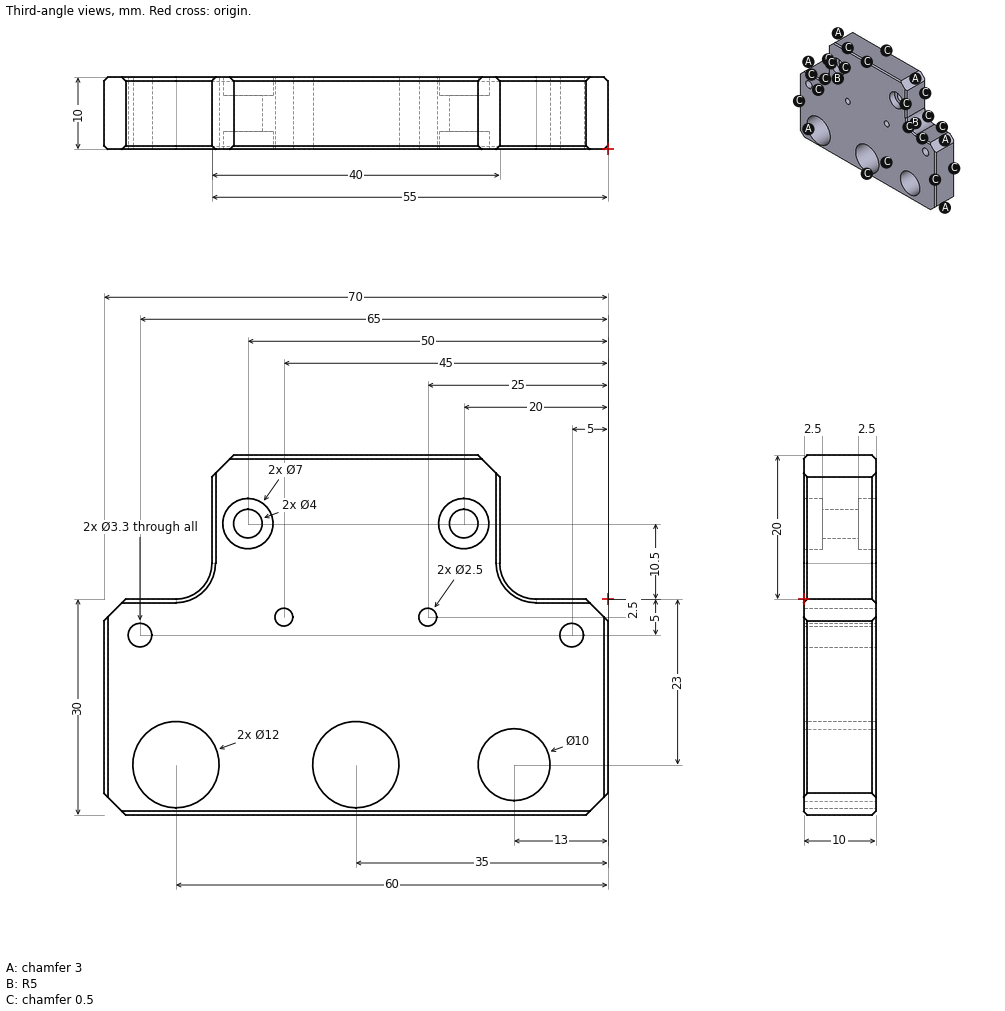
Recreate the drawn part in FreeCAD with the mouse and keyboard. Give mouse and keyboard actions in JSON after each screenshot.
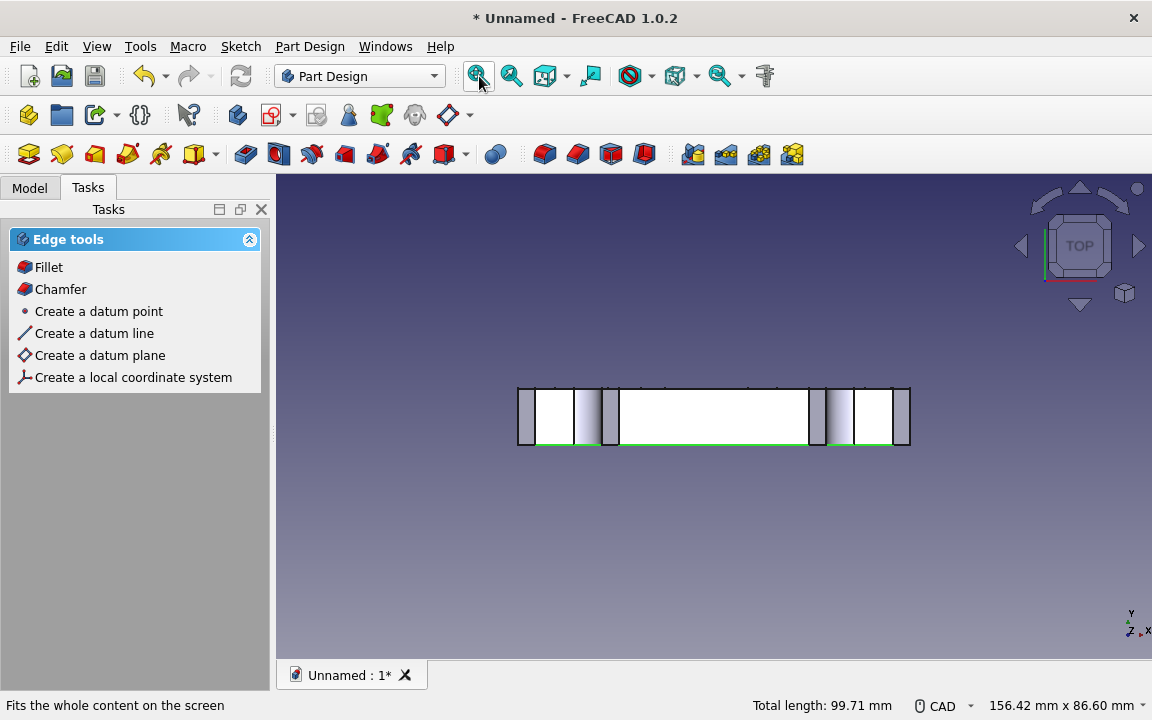
{"action": "left_click", "coordinate": [874, 387], "text": "ctrl"}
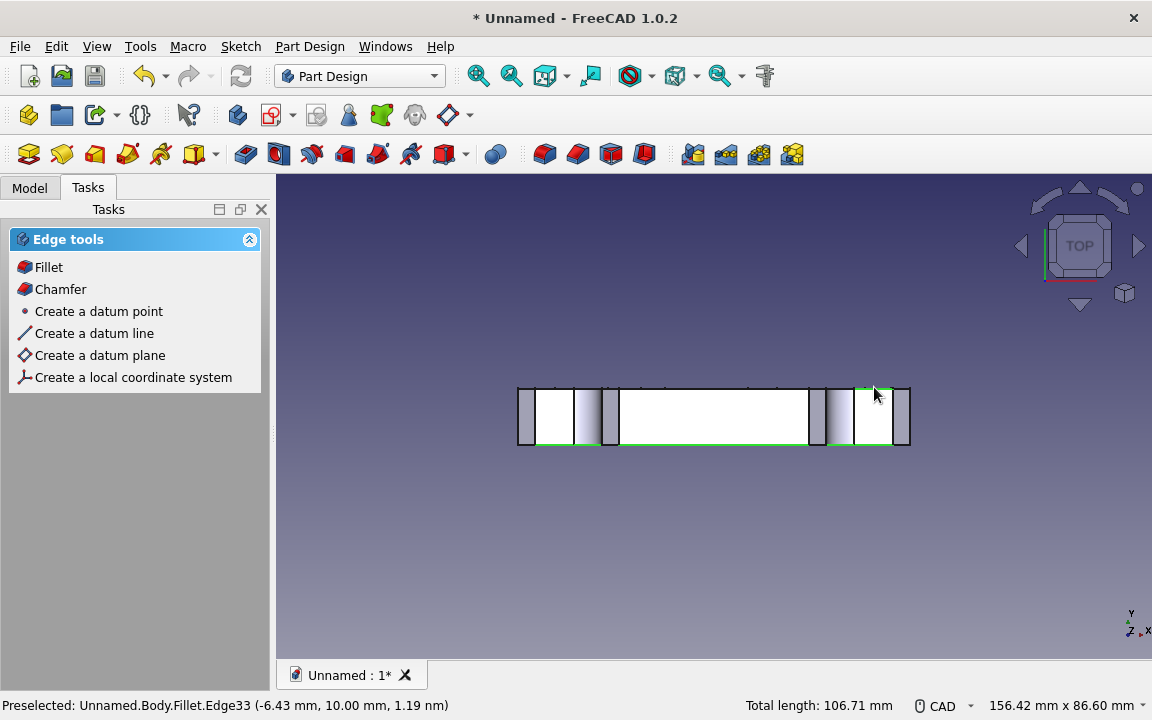
{"action": "left_click", "coordinate": [834, 387], "text": "ctrl"}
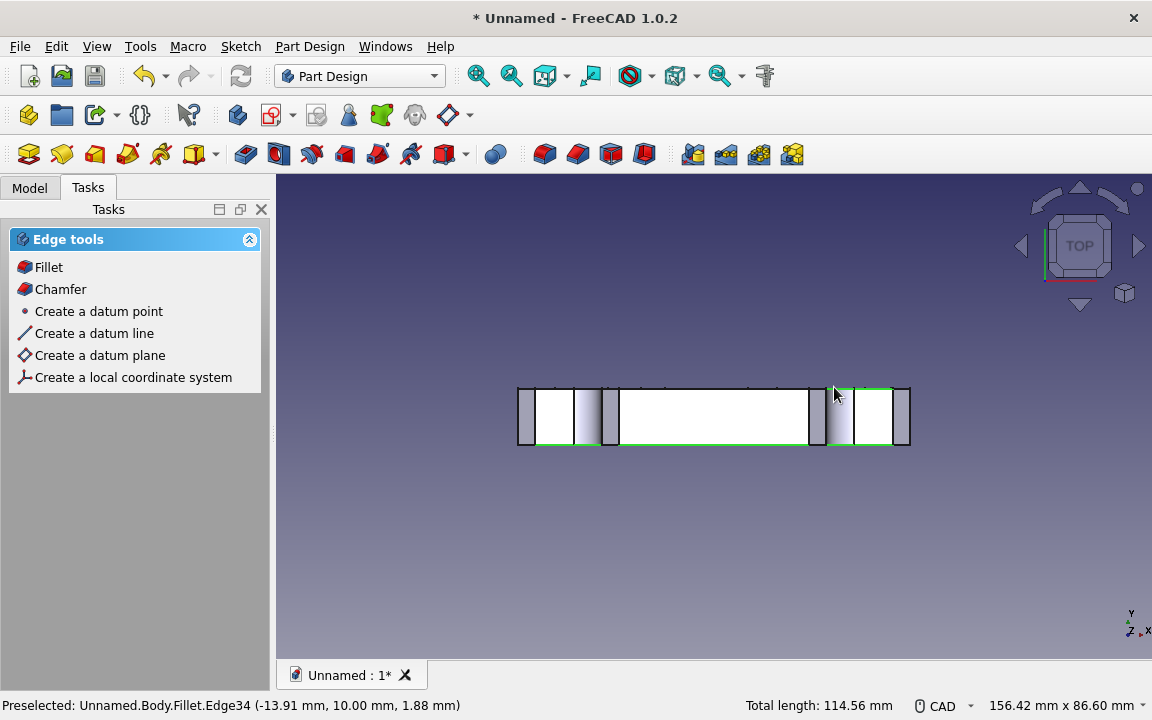
{"action": "left_click", "coordinate": [594, 387], "text": "ctrl"}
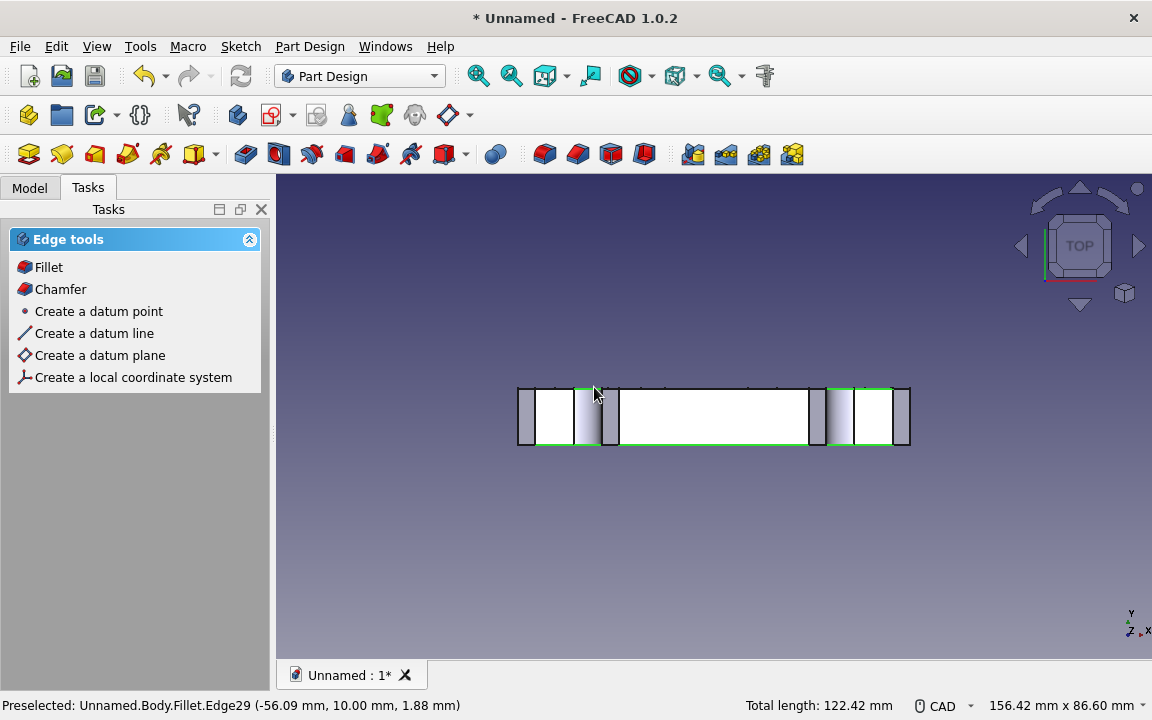
{"action": "left_click", "coordinate": [554, 387], "text": "ctrl"}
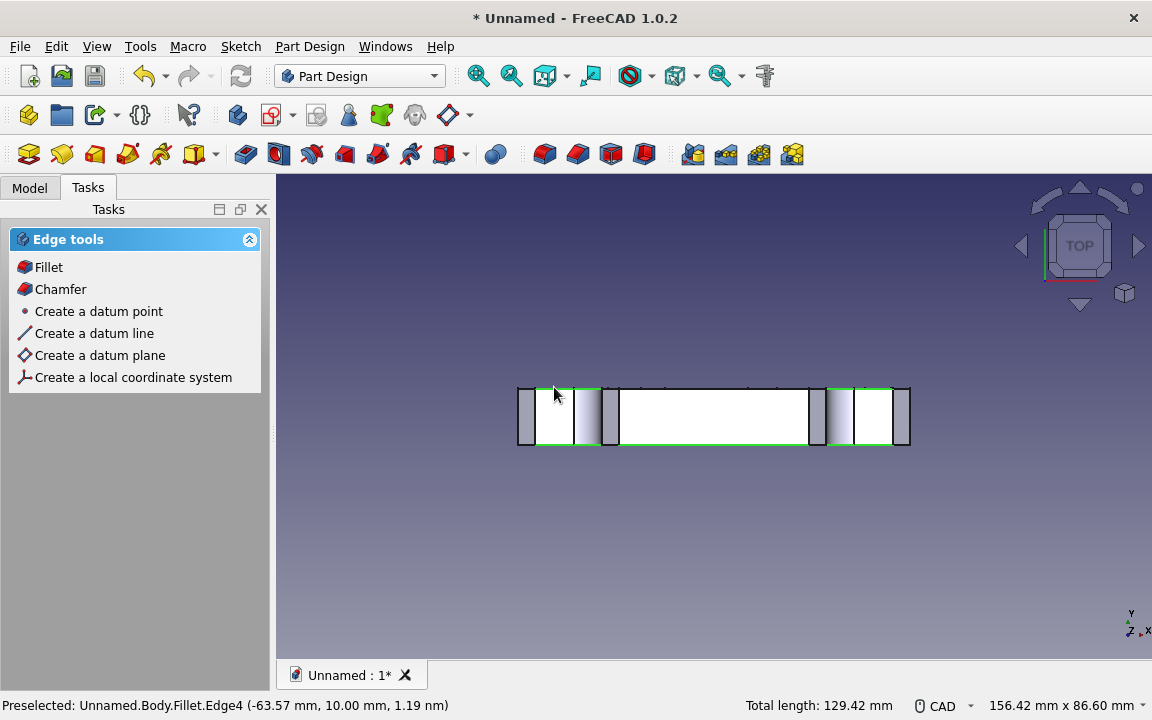
{"action": "left_click", "coordinate": [714, 387], "text": "ctrl"}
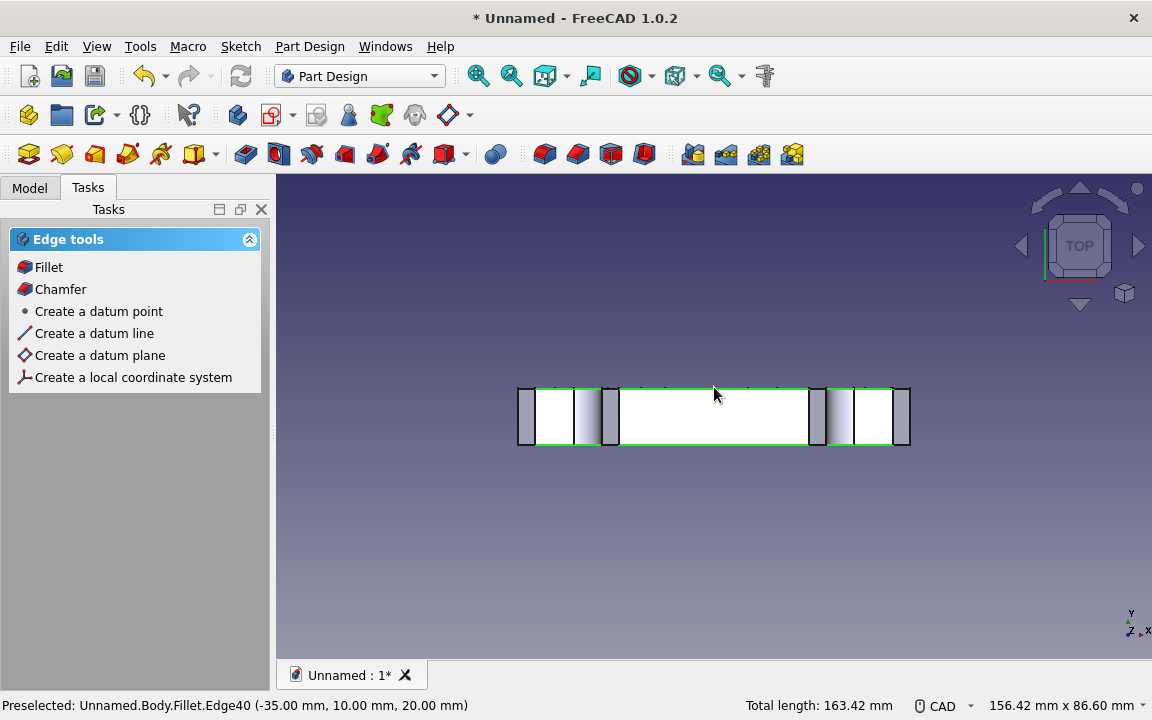
{"action": "key", "text": "0"}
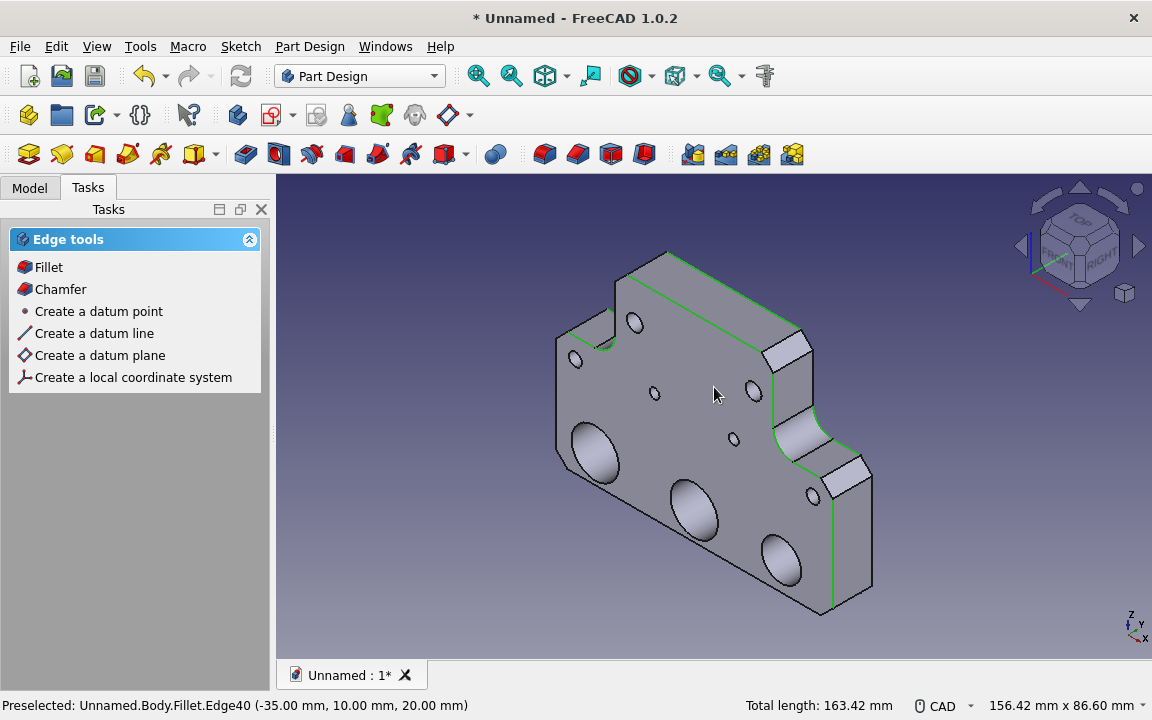
{"action": "key", "text": "1"}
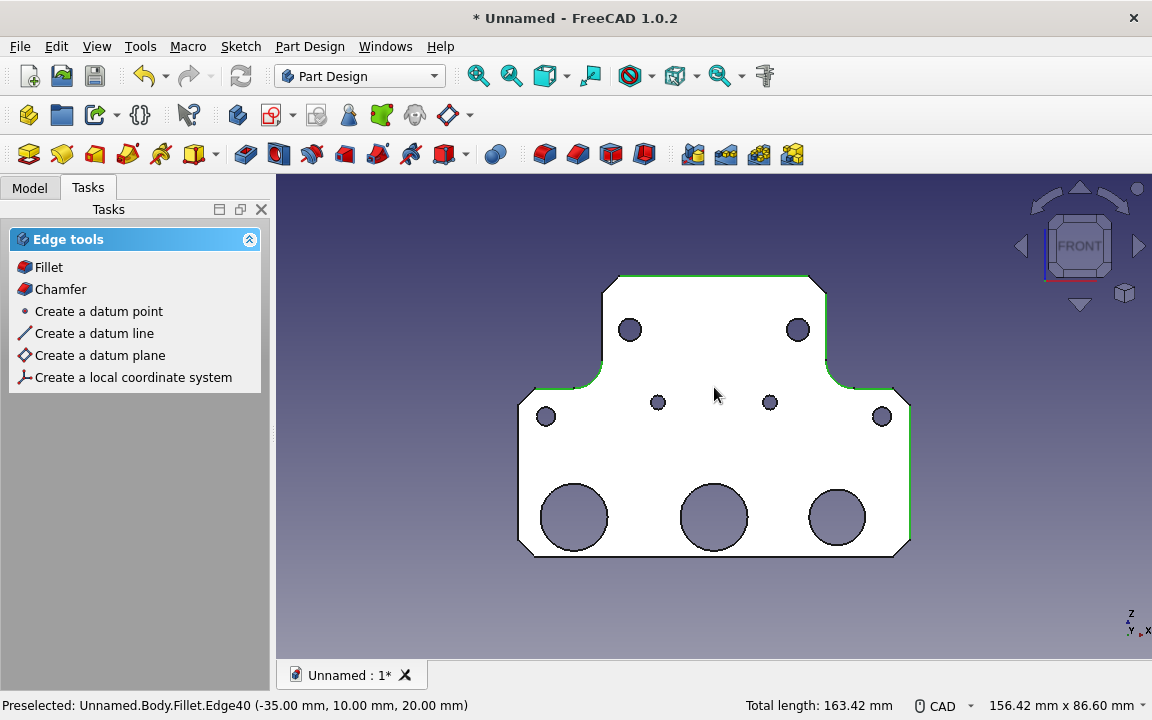
{"action": "left_click", "coordinate": [518, 485], "text": "ctrl"}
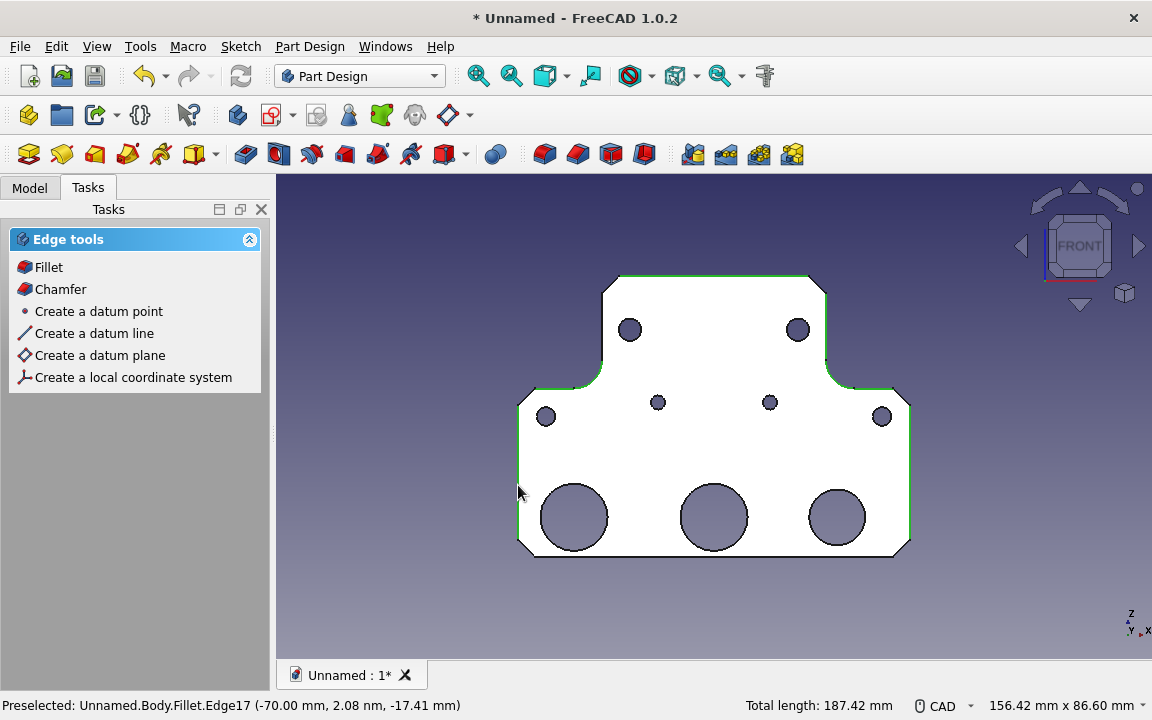
{"action": "key", "text": "3"}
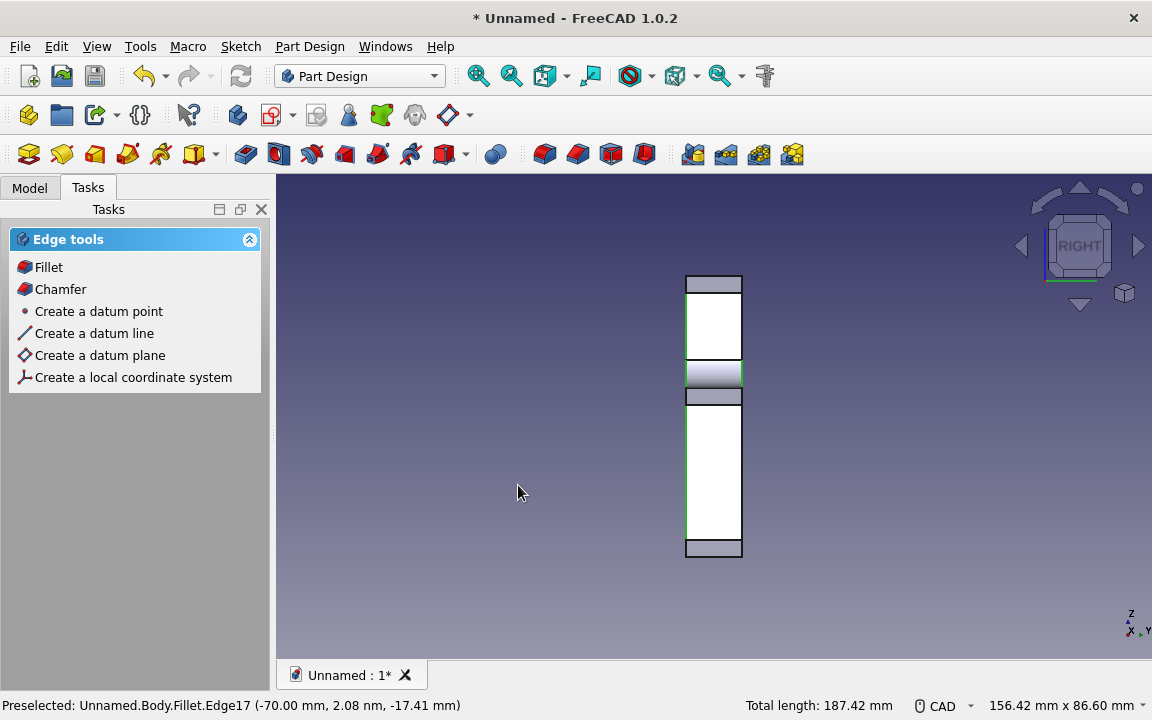
{"action": "left_click", "coordinate": [742, 458], "text": "ctrl"}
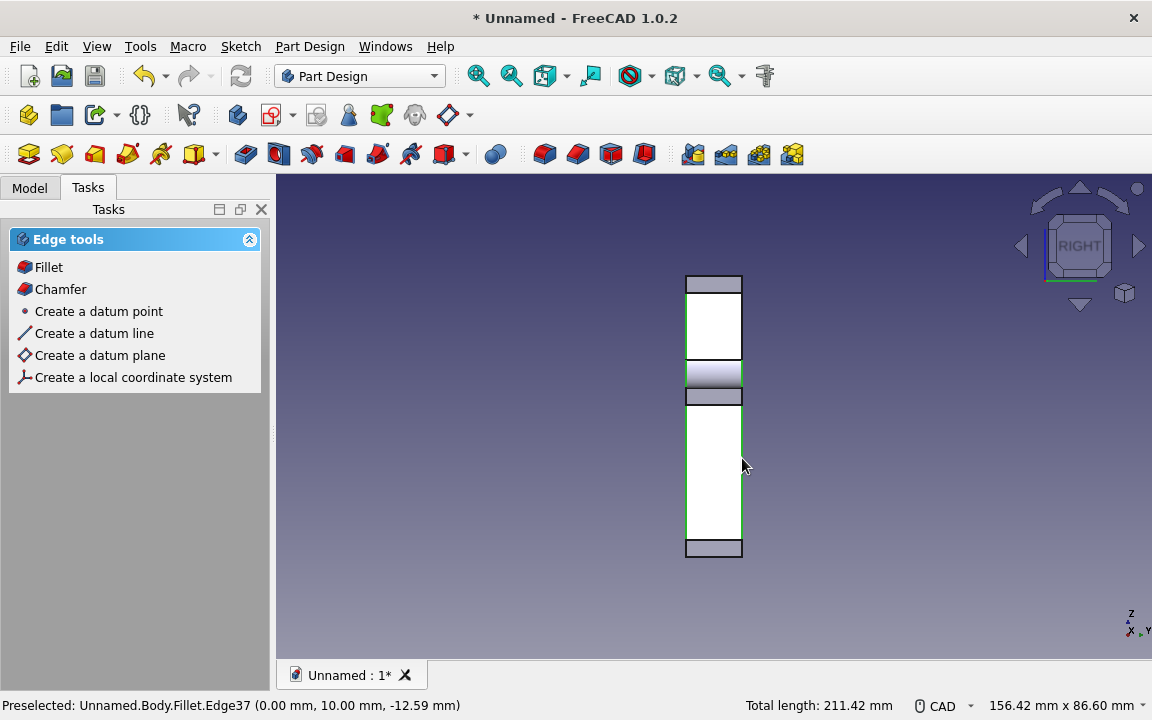
{"action": "left_click", "coordinate": [742, 326], "text": "ctrl"}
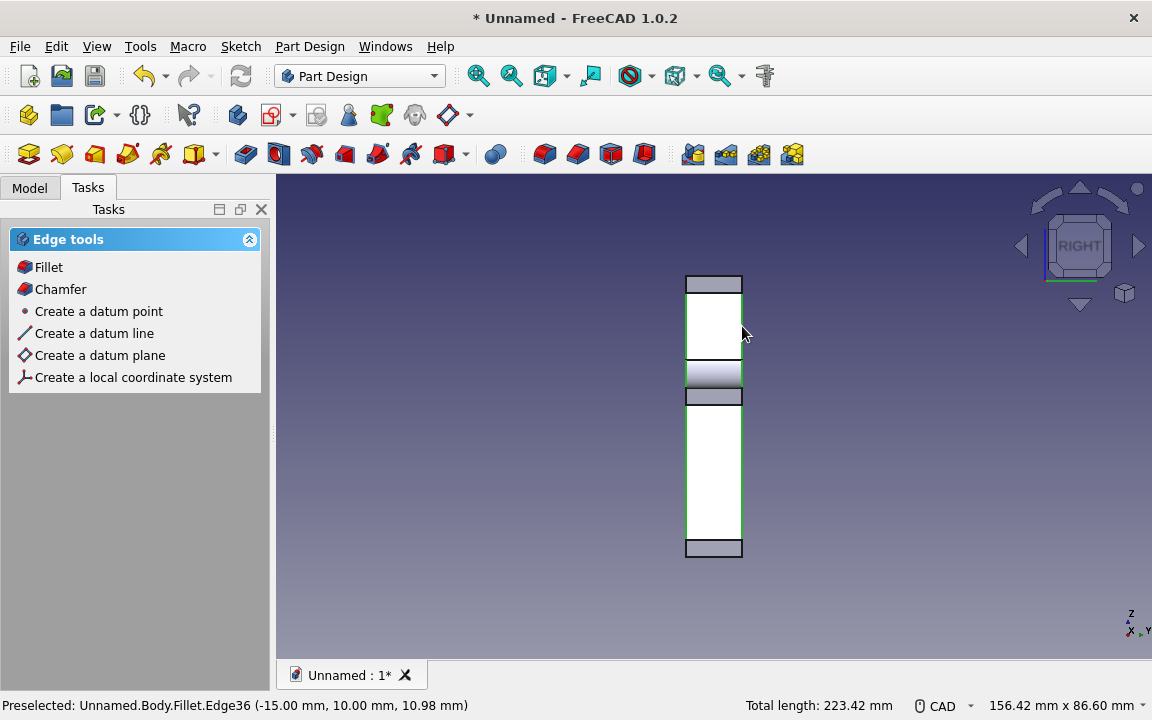
{"action": "key", "text": "5"}